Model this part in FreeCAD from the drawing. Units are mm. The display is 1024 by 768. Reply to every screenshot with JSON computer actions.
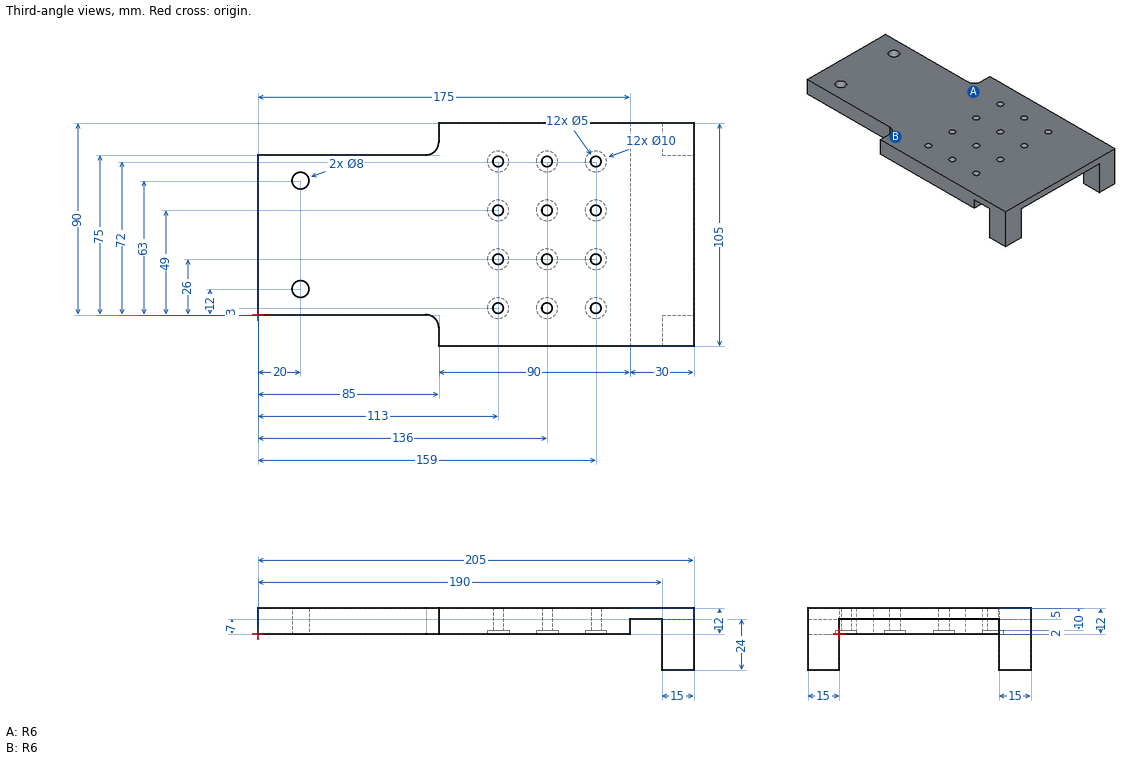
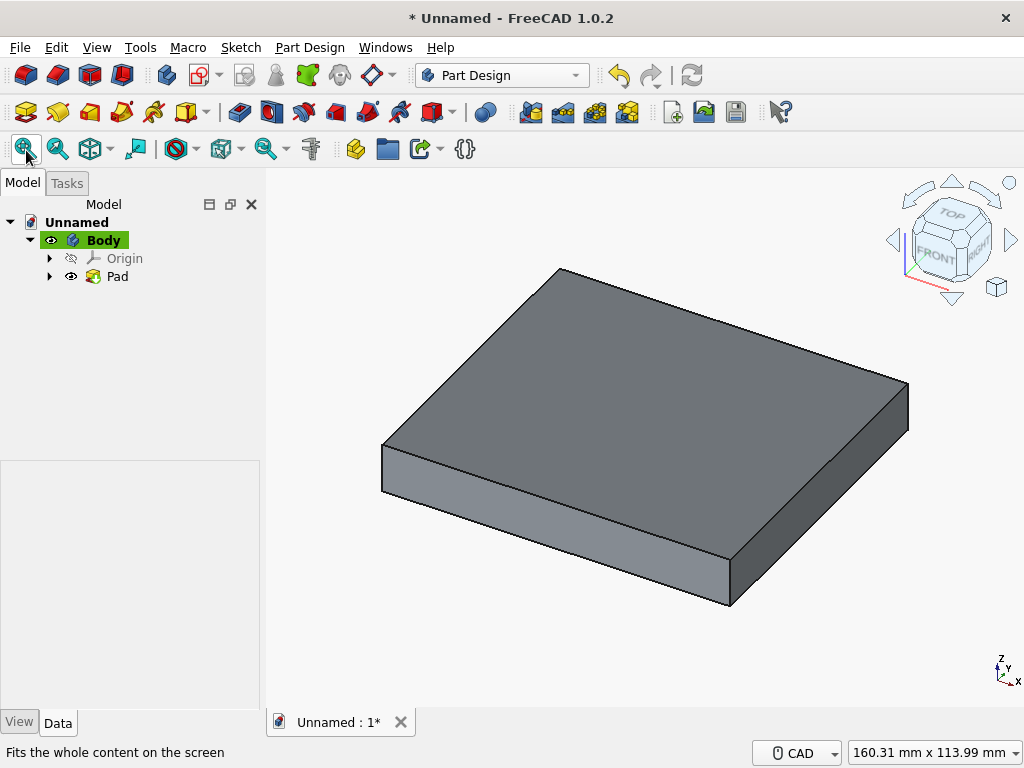
{"action": "left_click", "coordinate": [645, 413]}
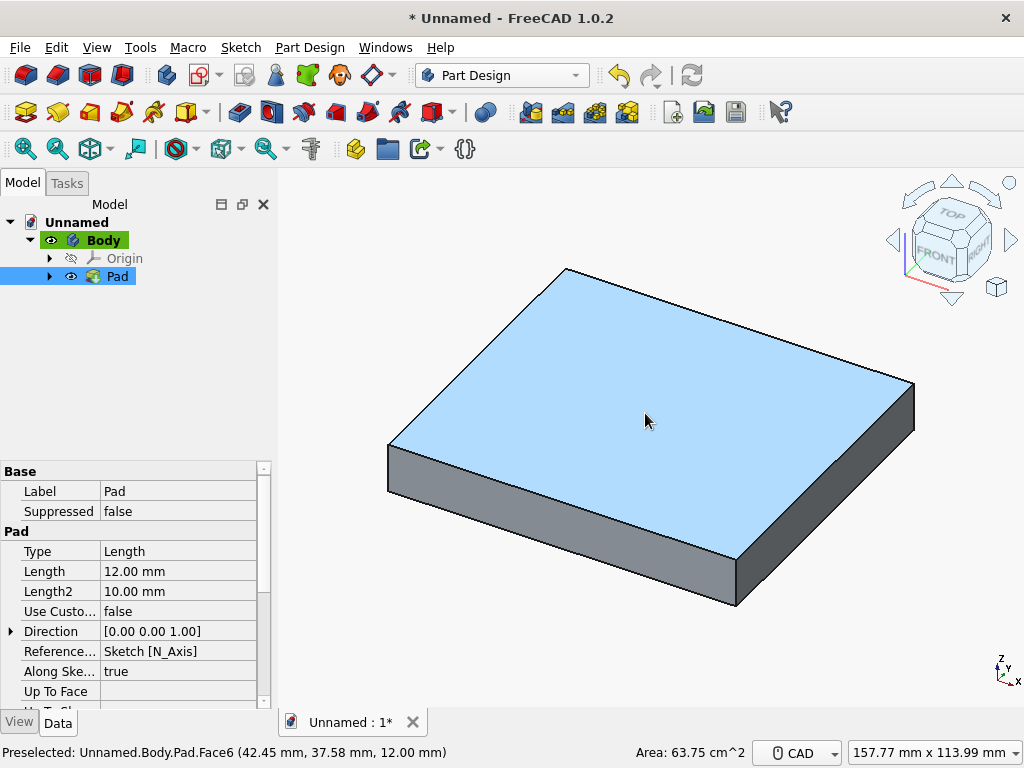
{"action": "left_click", "coordinate": [200, 76]}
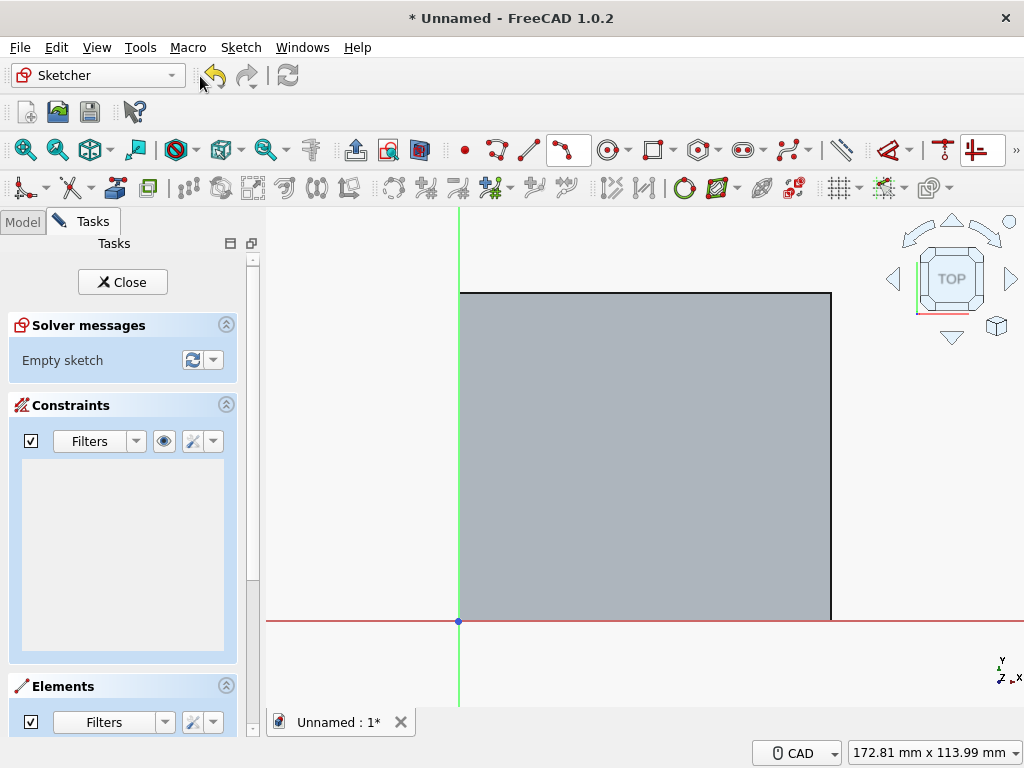
{"action": "scroll", "coordinate": [294, 457], "scroll_direction": "down", "scroll_amount": 3}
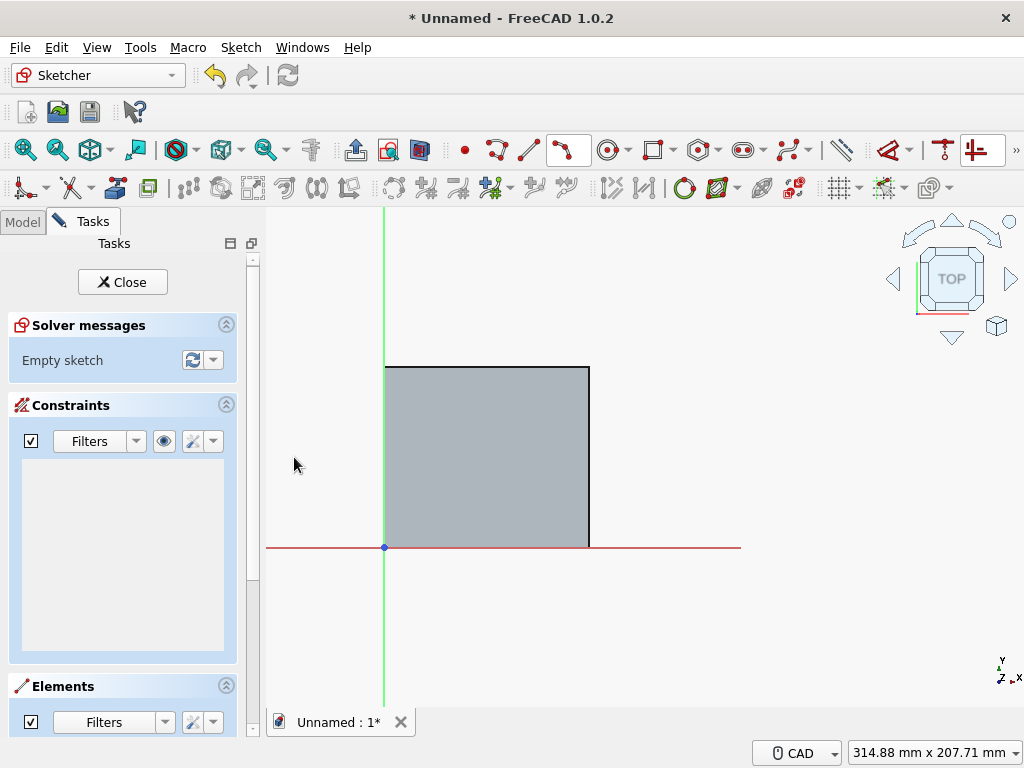
{"action": "key", "text": "g r"}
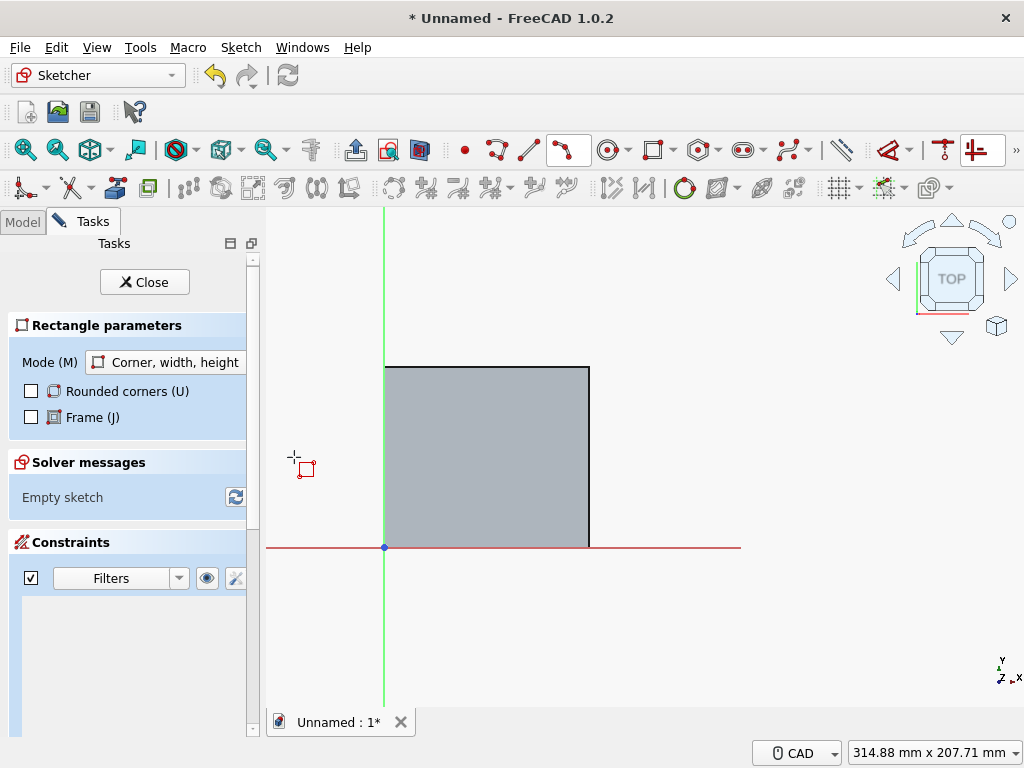
{"action": "left_click", "coordinate": [589, 331]}
{"action": "mouse_move", "coordinate": [806, 584]}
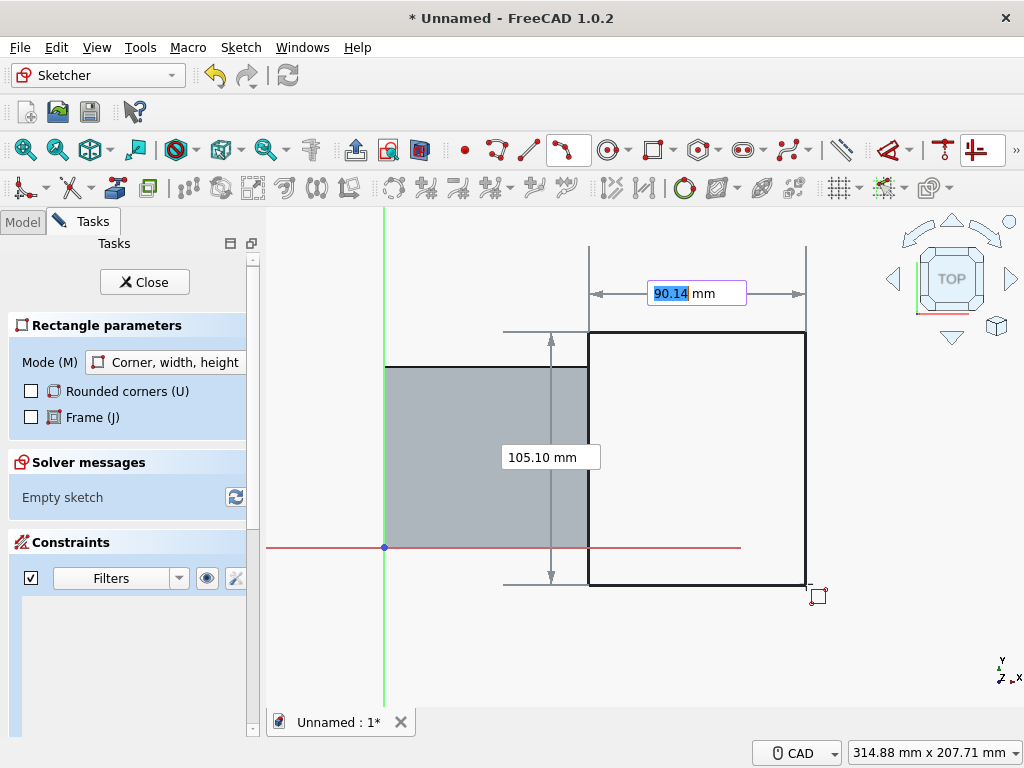
{"action": "type", "text": "90"}
{"action": "key", "text": "Tab"}
{"action": "type", "text": "105"}
{"action": "key", "text": "Return"}
{"action": "key", "text": "Escape"}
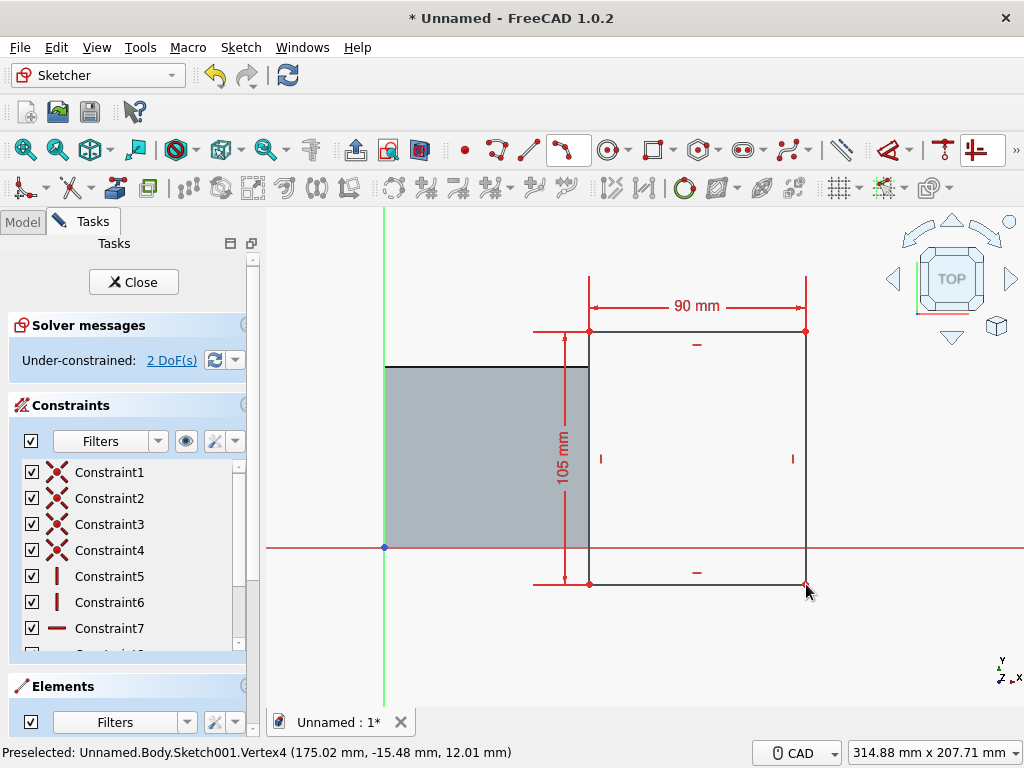
{"action": "left_click", "coordinate": [888, 150]}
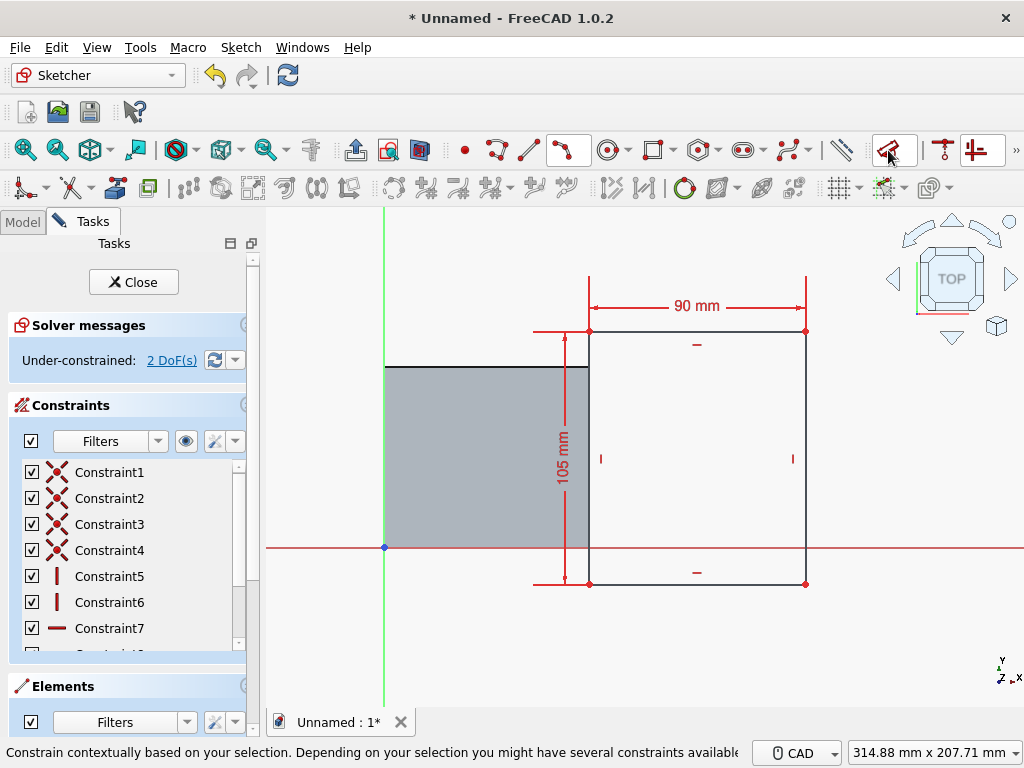
{"action": "left_click", "coordinate": [589, 332]}
{"action": "left_click", "coordinate": [487, 298]}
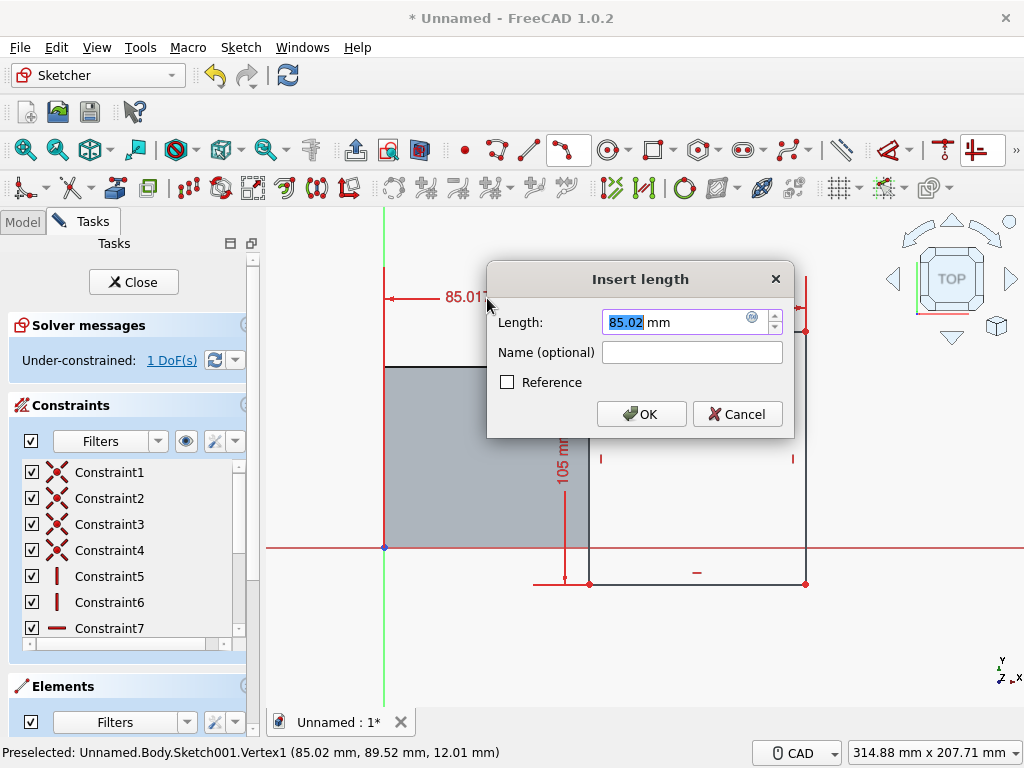
{"action": "type", "text": "85"}
{"action": "key", "text": "Return"}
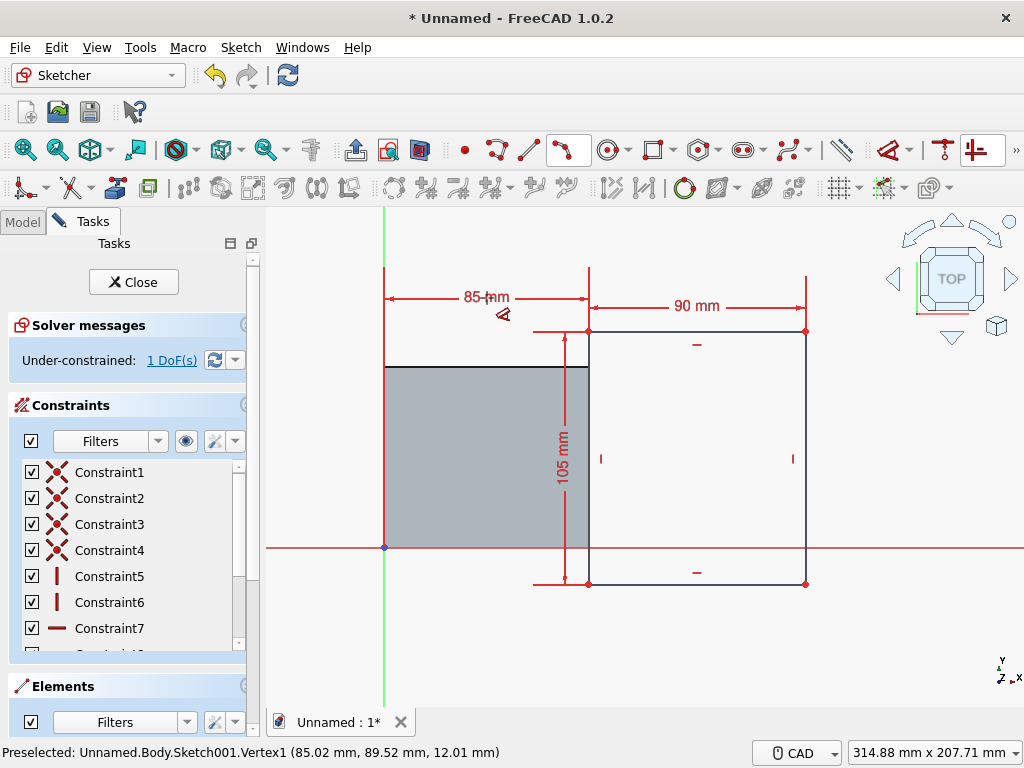
{"action": "left_click", "coordinate": [589, 332]}
{"action": "left_click", "coordinate": [350, 440]}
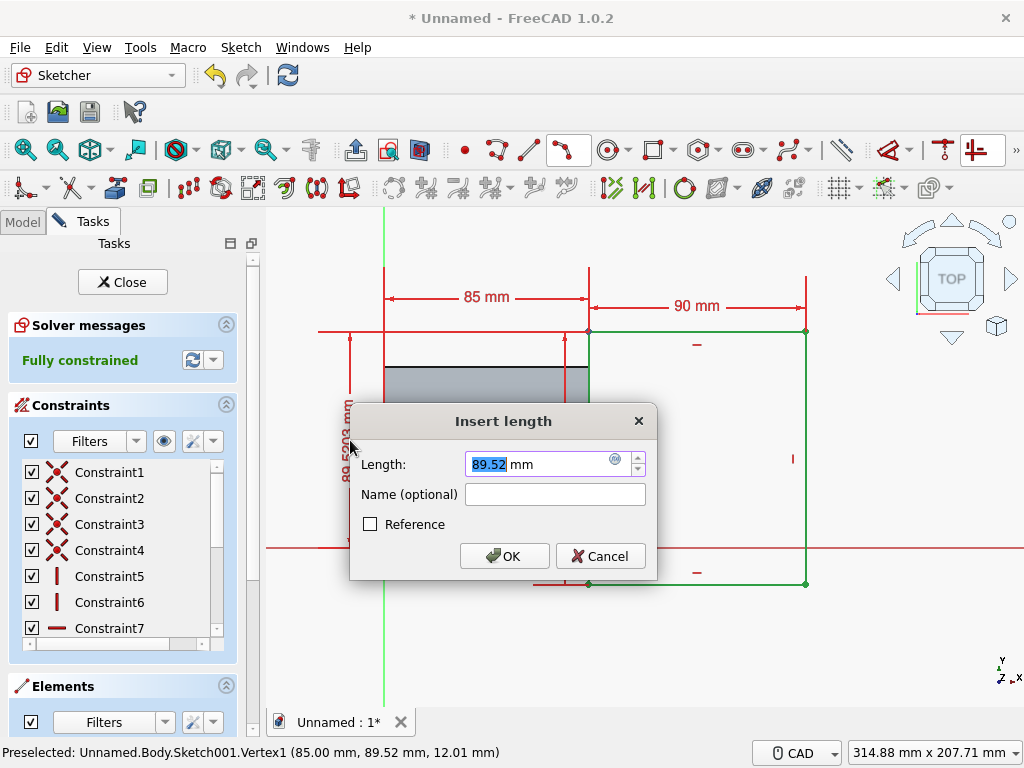
{"action": "type", "text": "90"}
{"action": "key", "text": "Return"}
{"action": "key", "text": "Escape"}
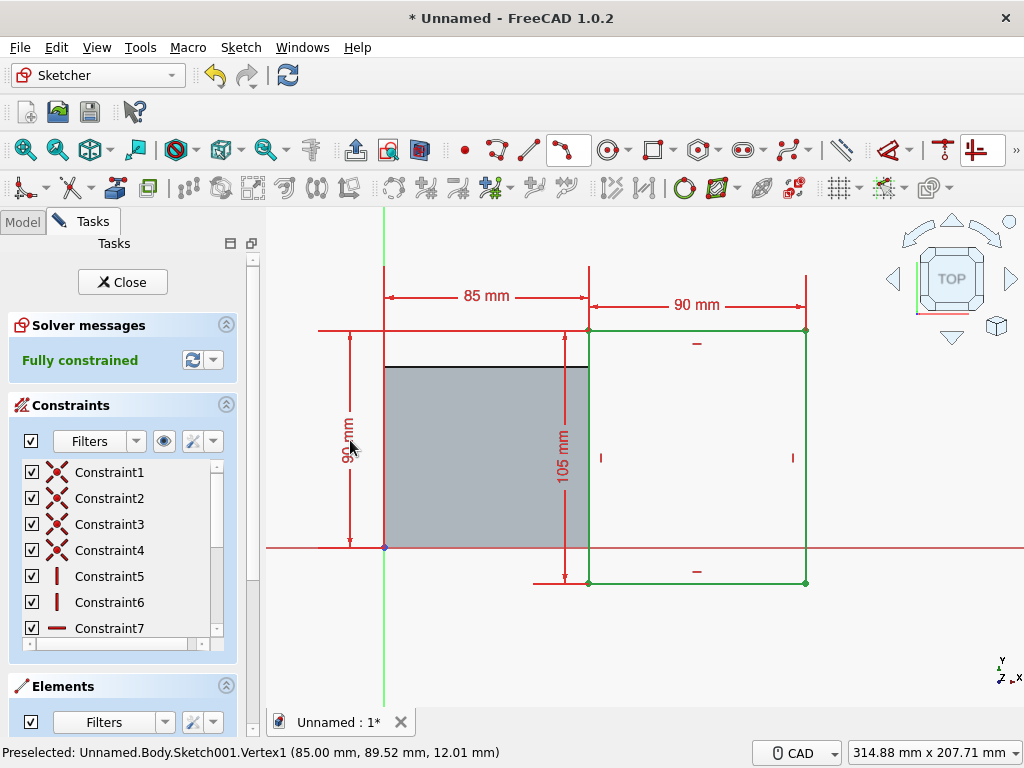
{"action": "left_click", "coordinate": [123, 282]}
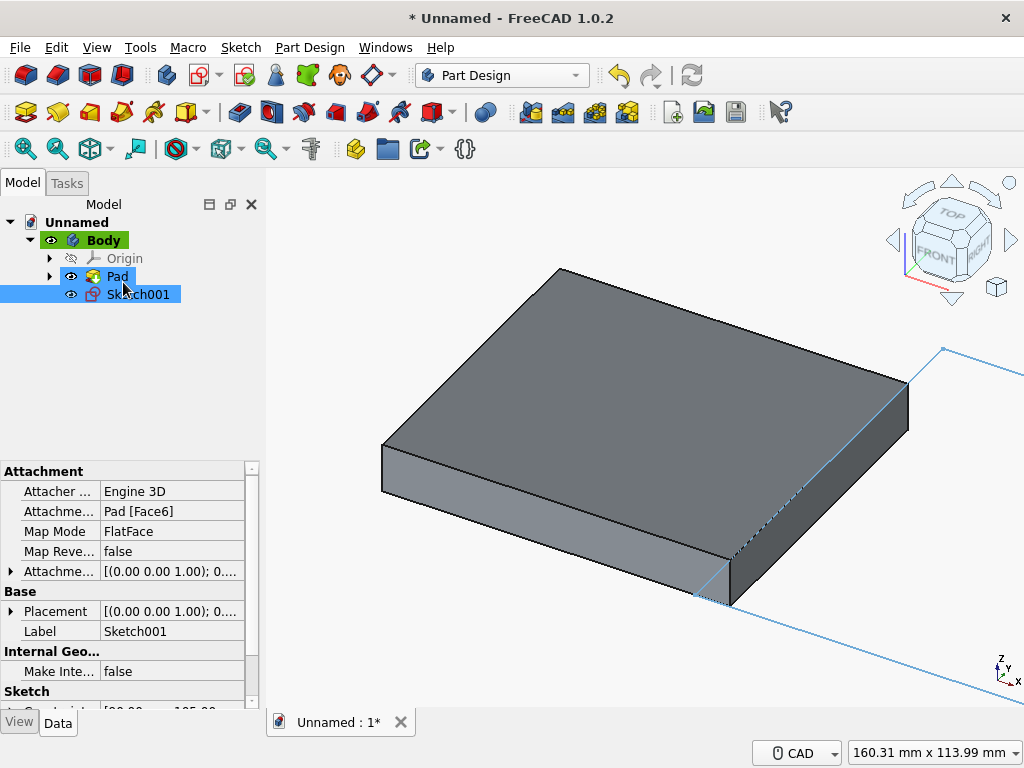
{"action": "left_click", "coordinate": [26, 112]}